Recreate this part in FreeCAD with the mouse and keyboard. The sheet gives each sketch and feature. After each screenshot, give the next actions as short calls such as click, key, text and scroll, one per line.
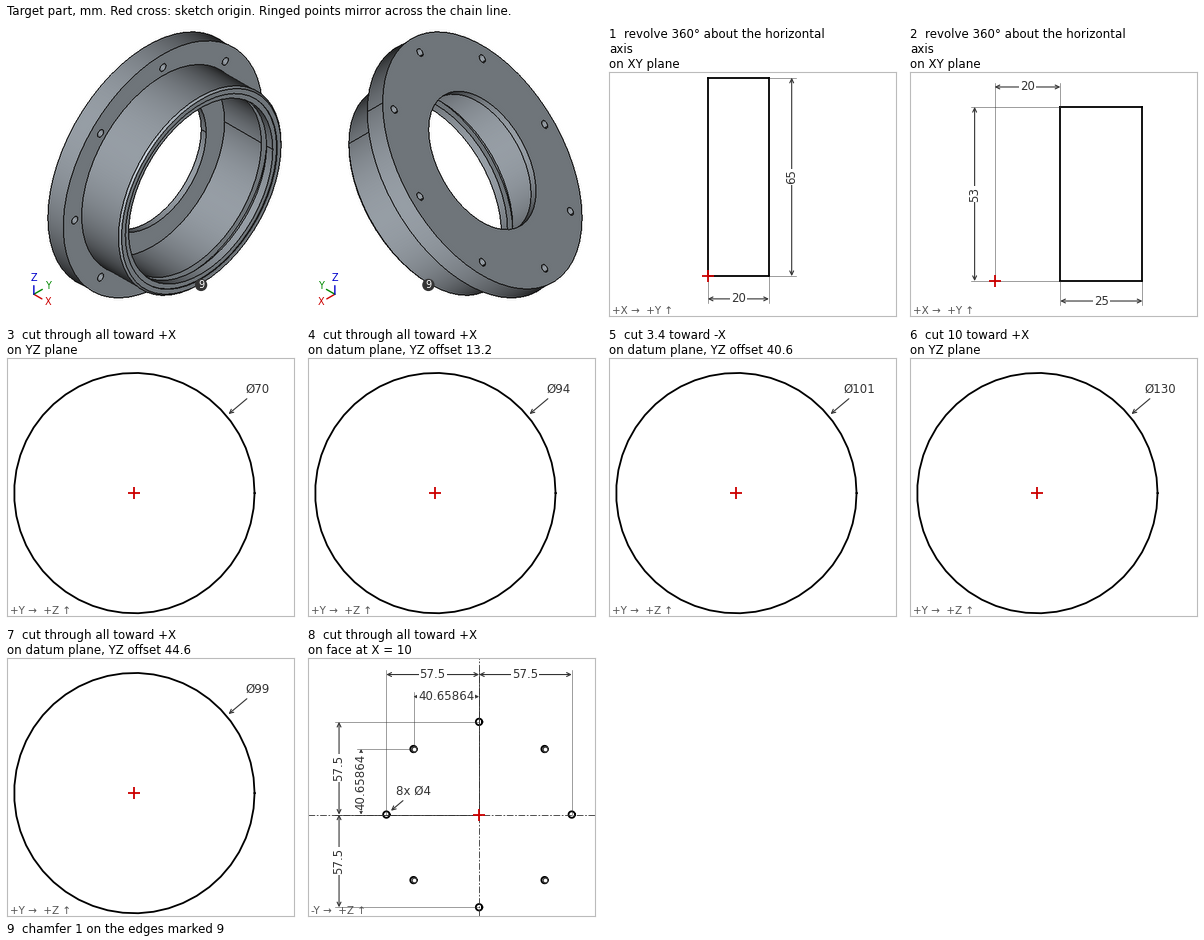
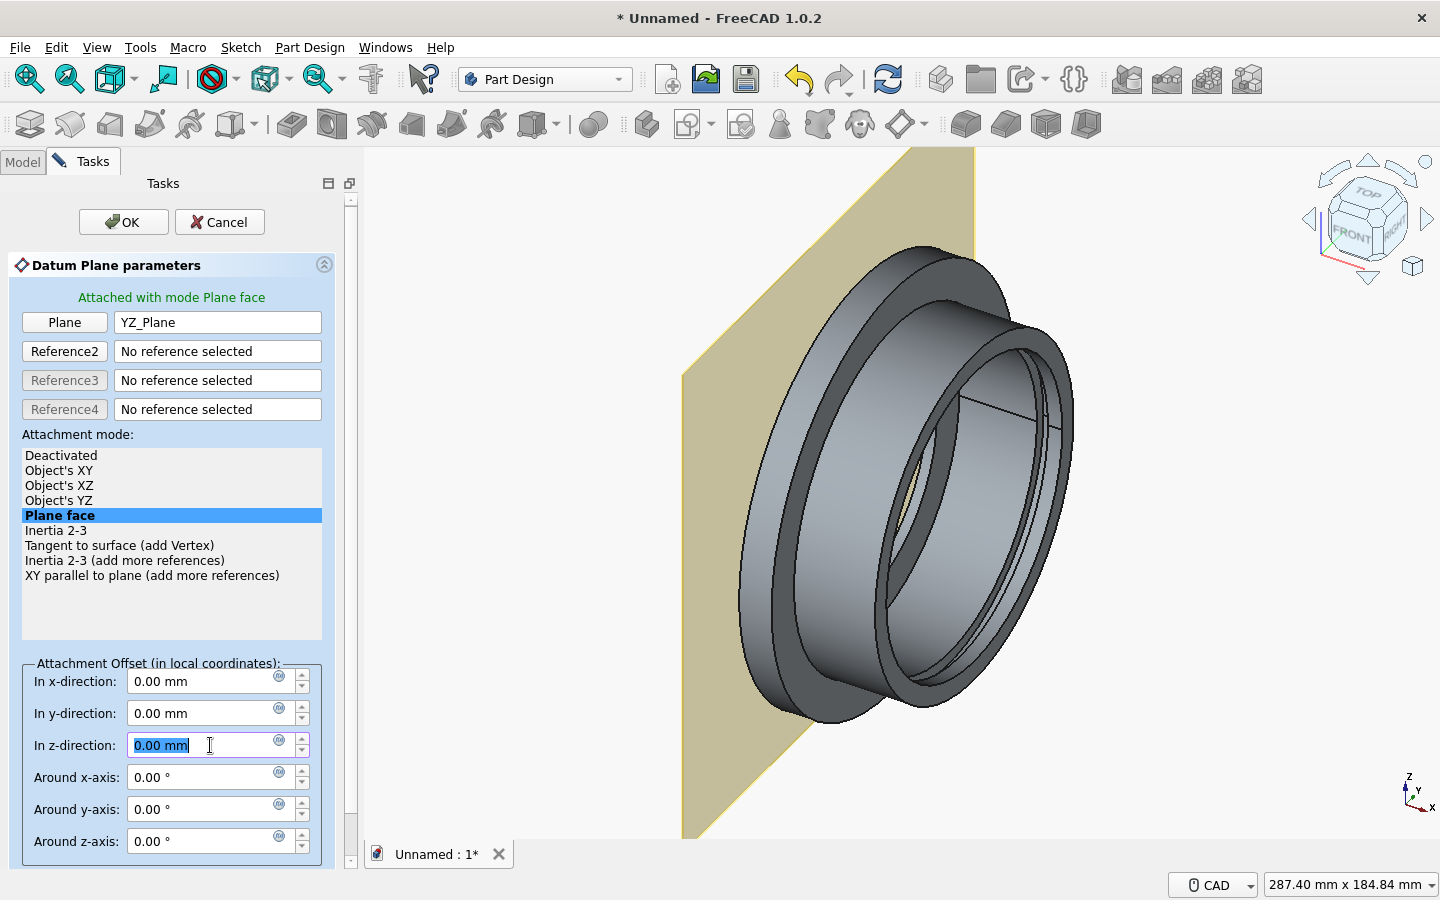
text(44.6)
key(Tab)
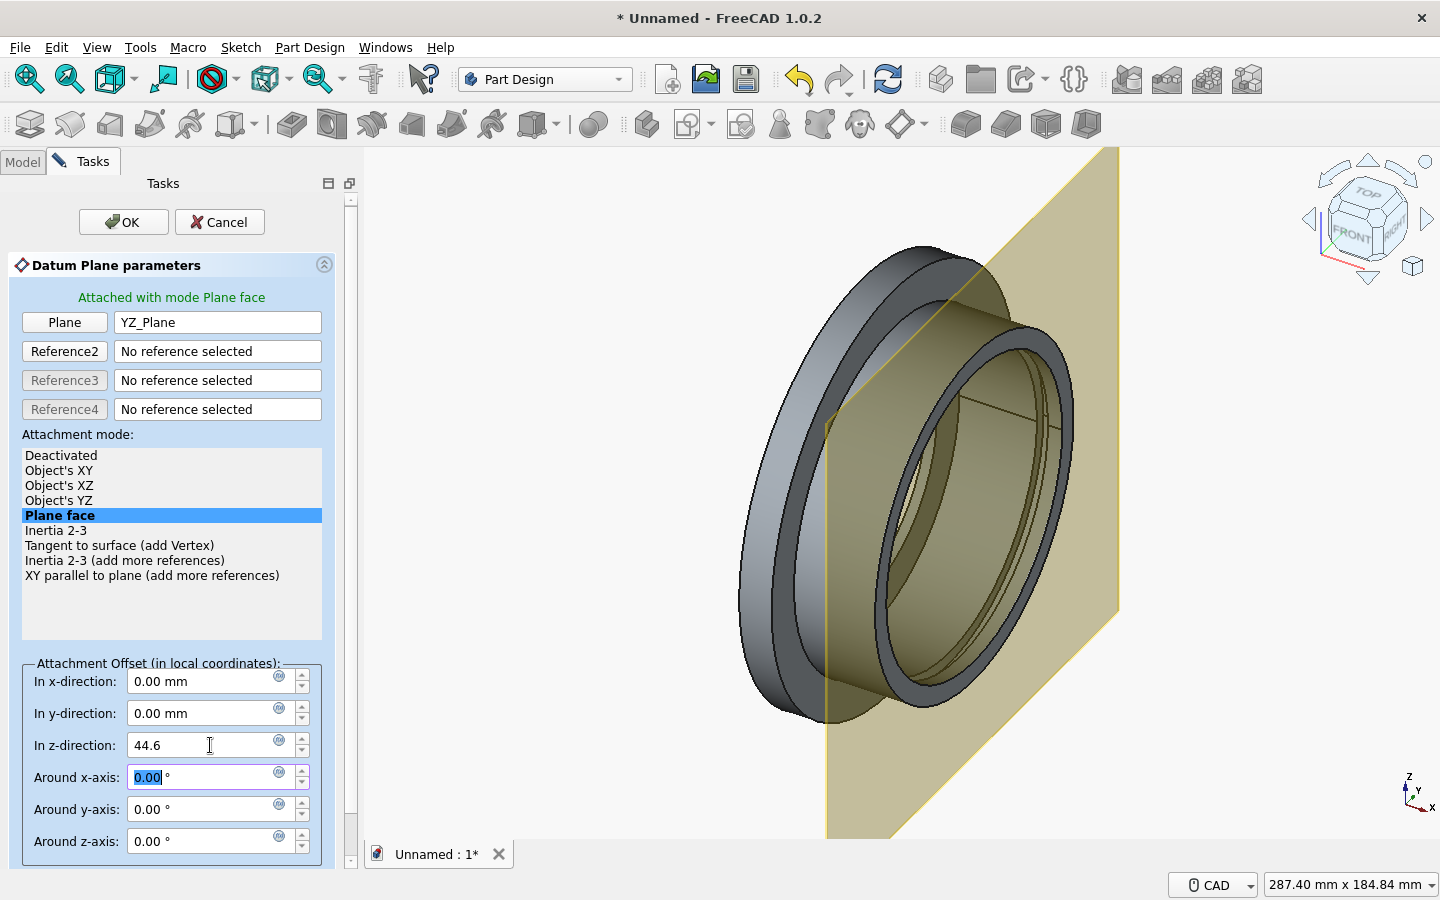
click(124, 222)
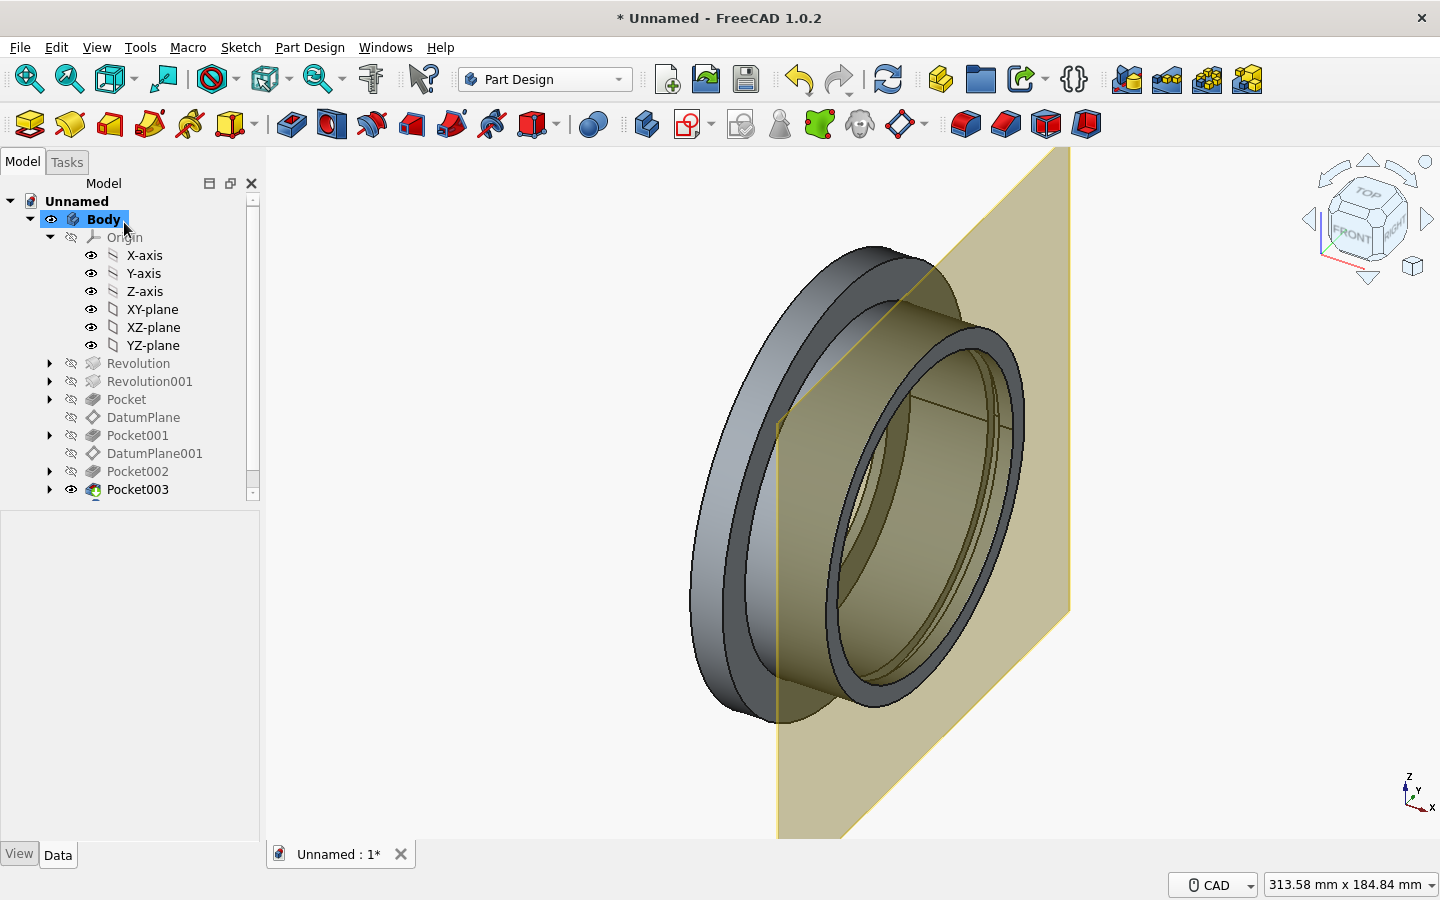
scroll(100, 341, down, 3)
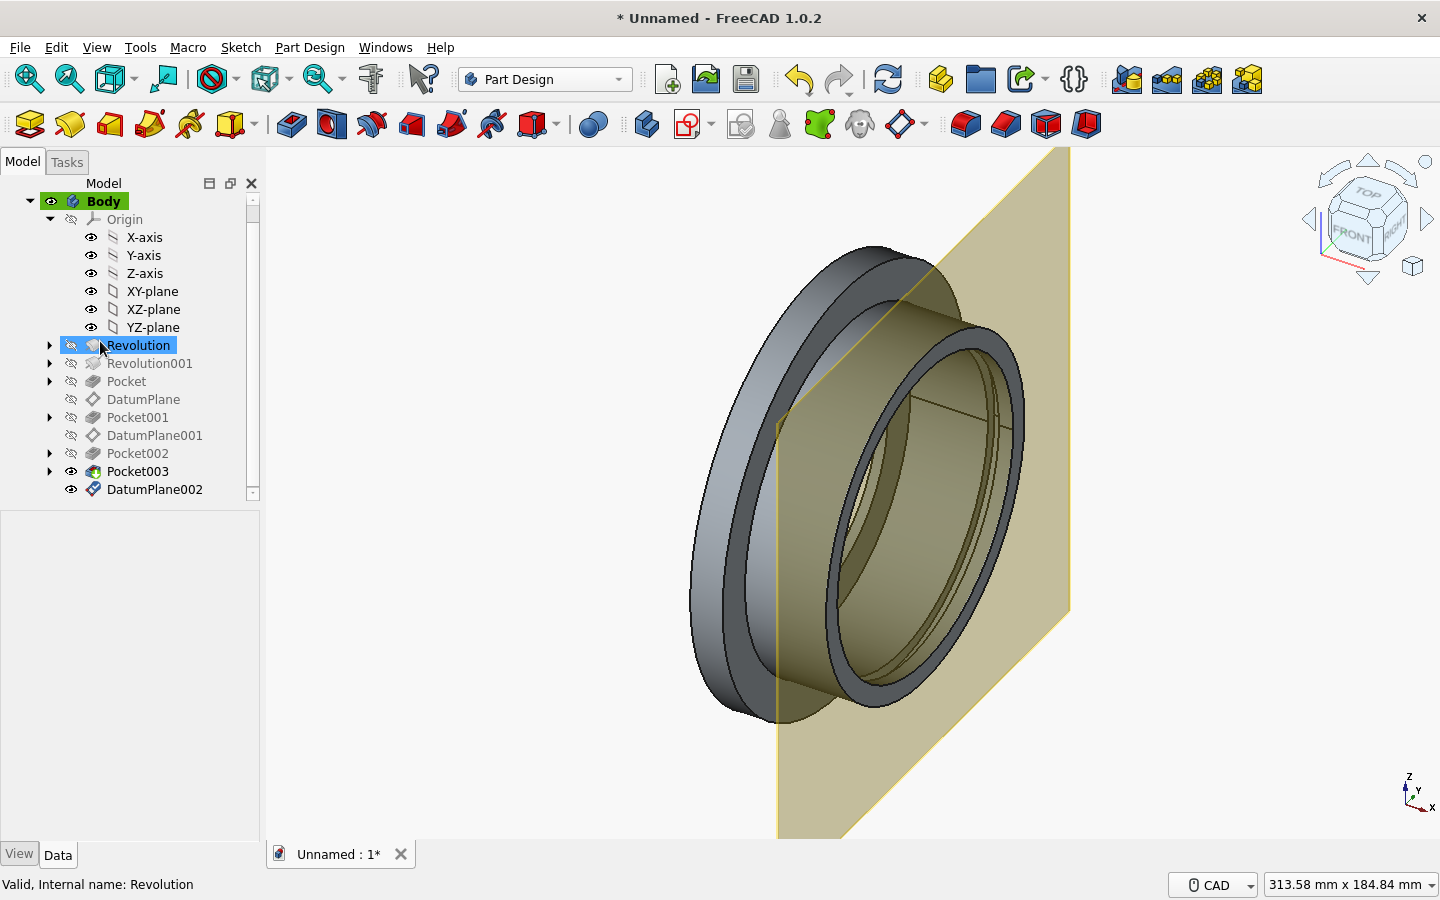
click(116, 489)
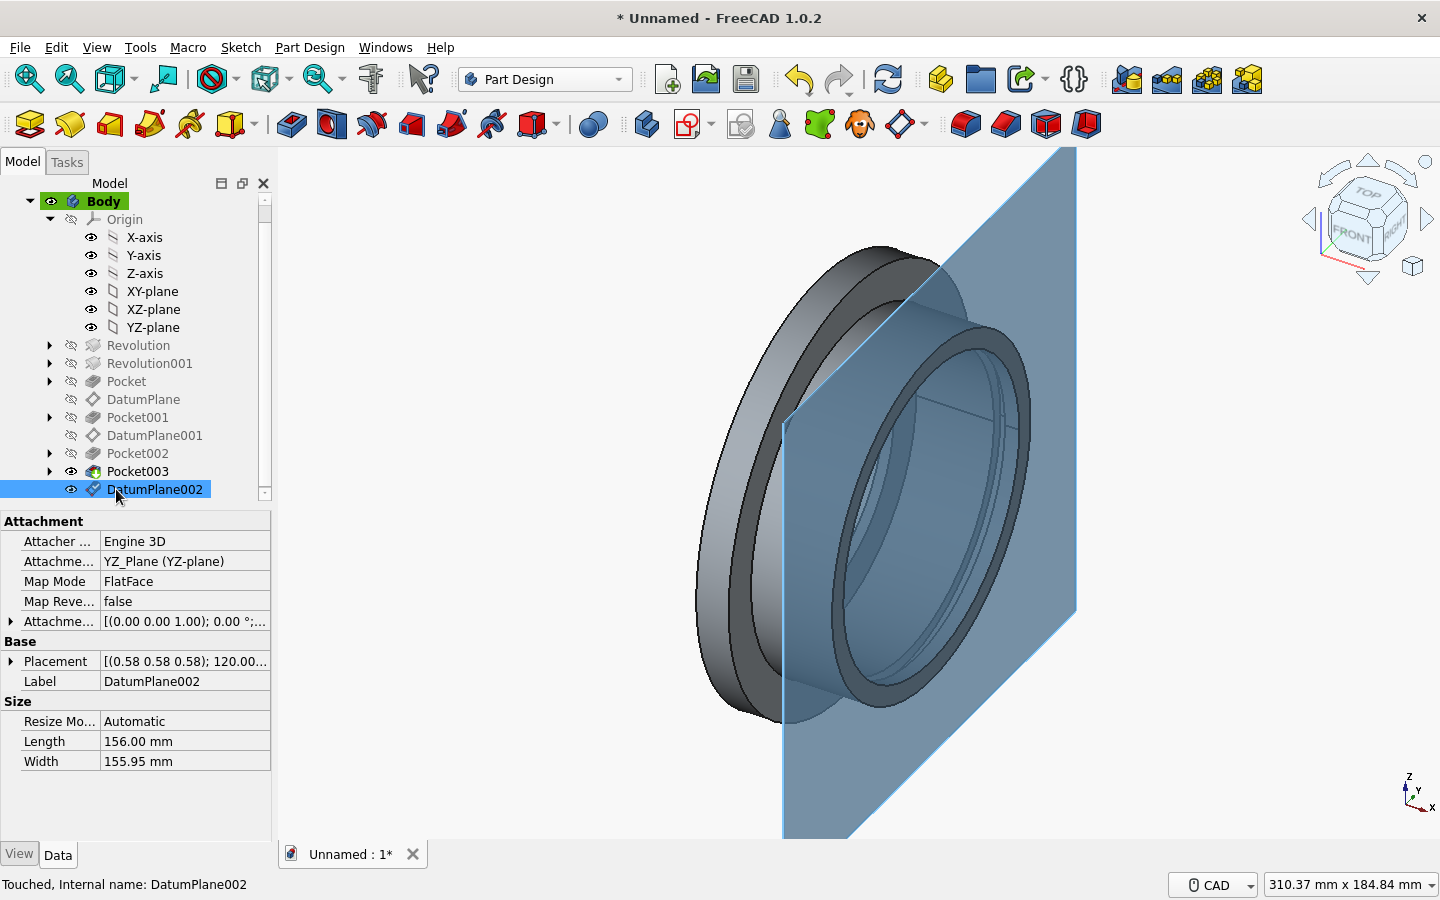
click(688, 124)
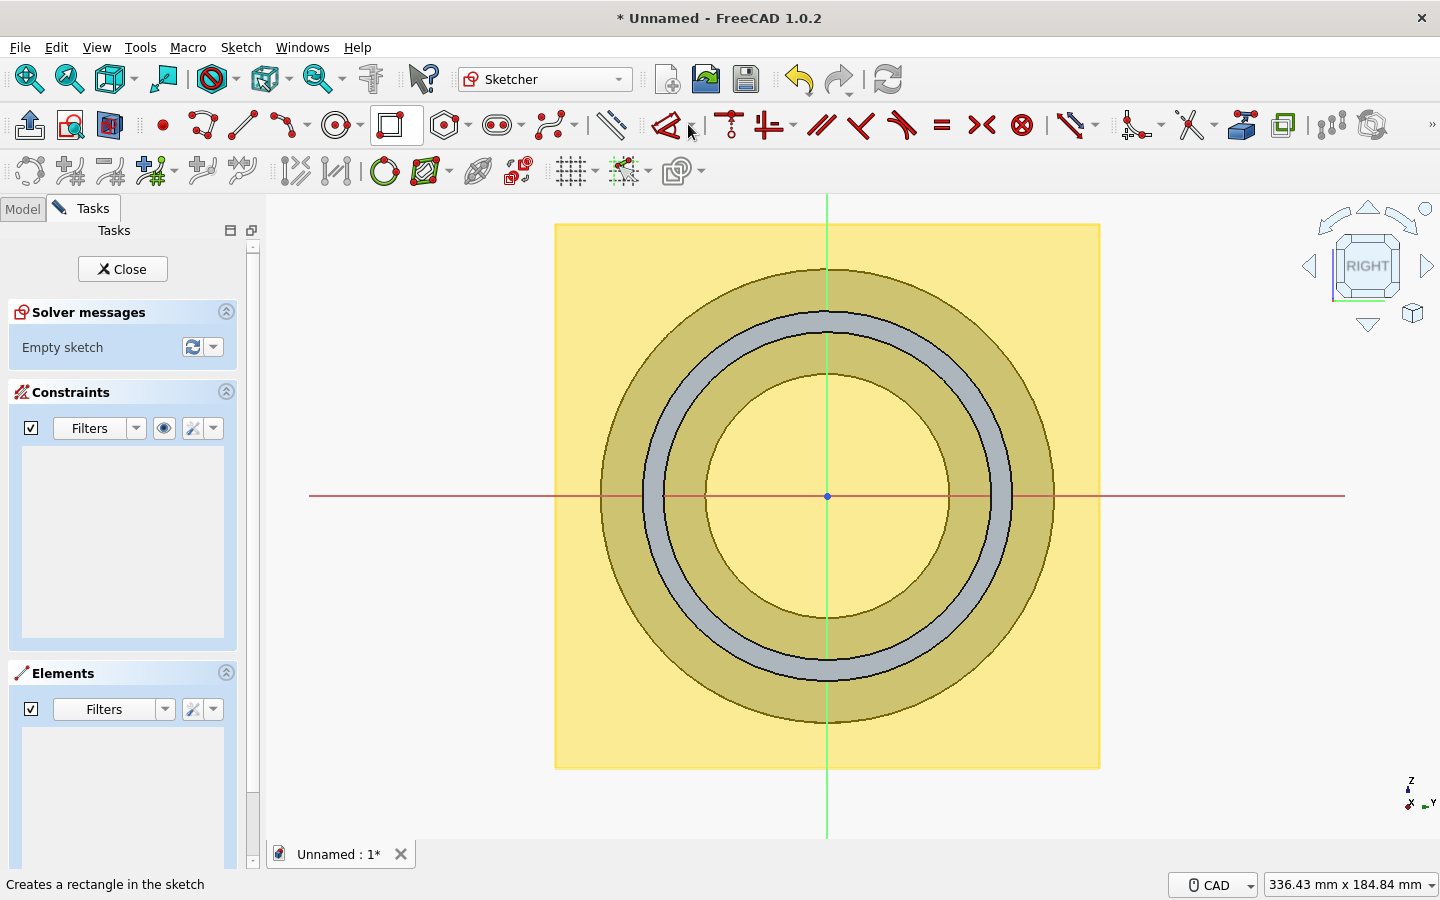
click(110, 126)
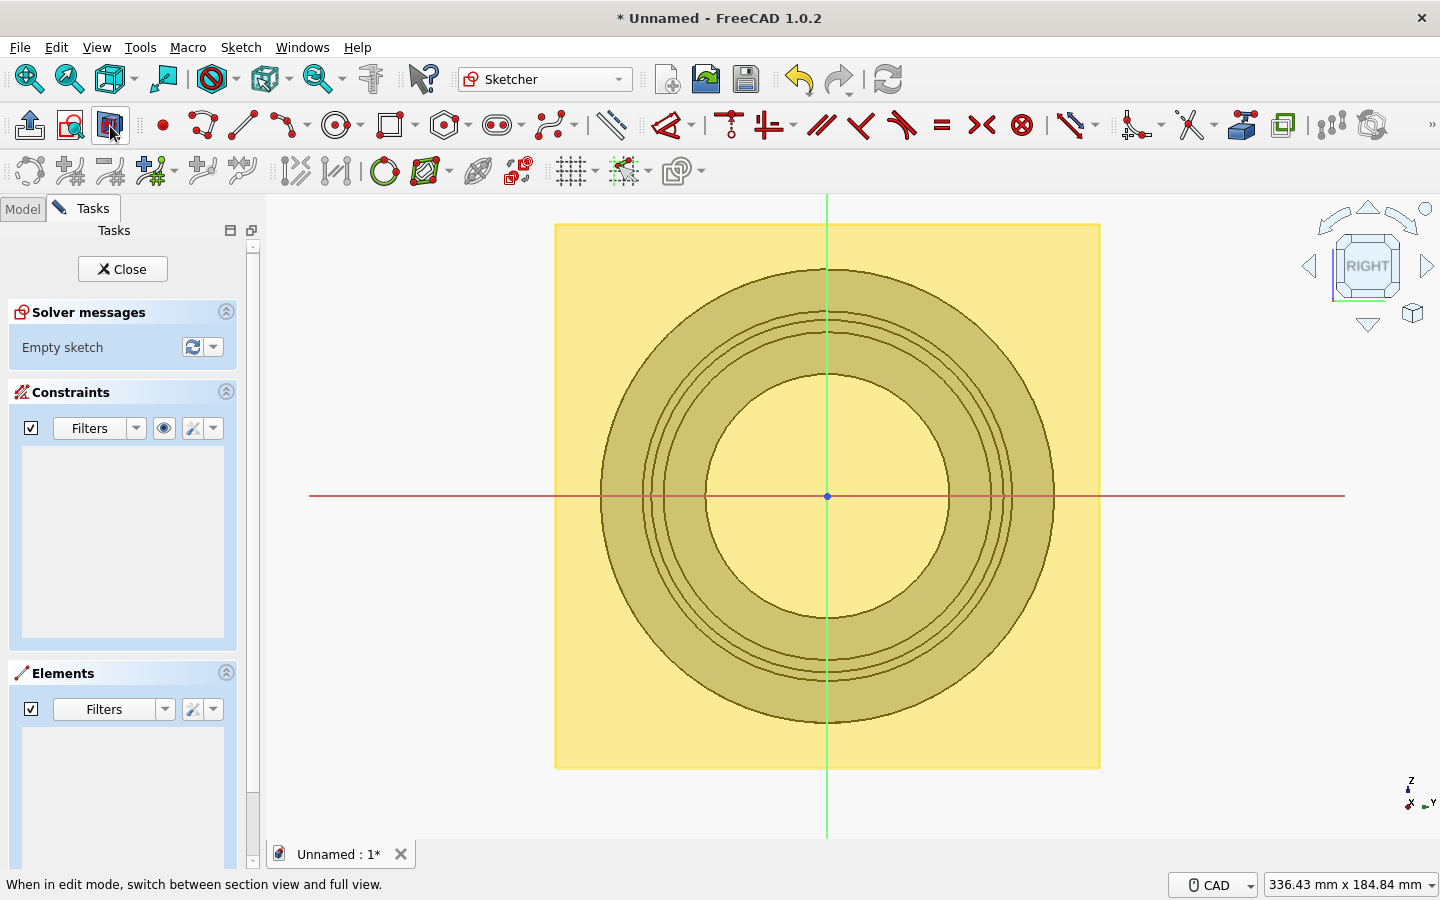
click(336, 126)